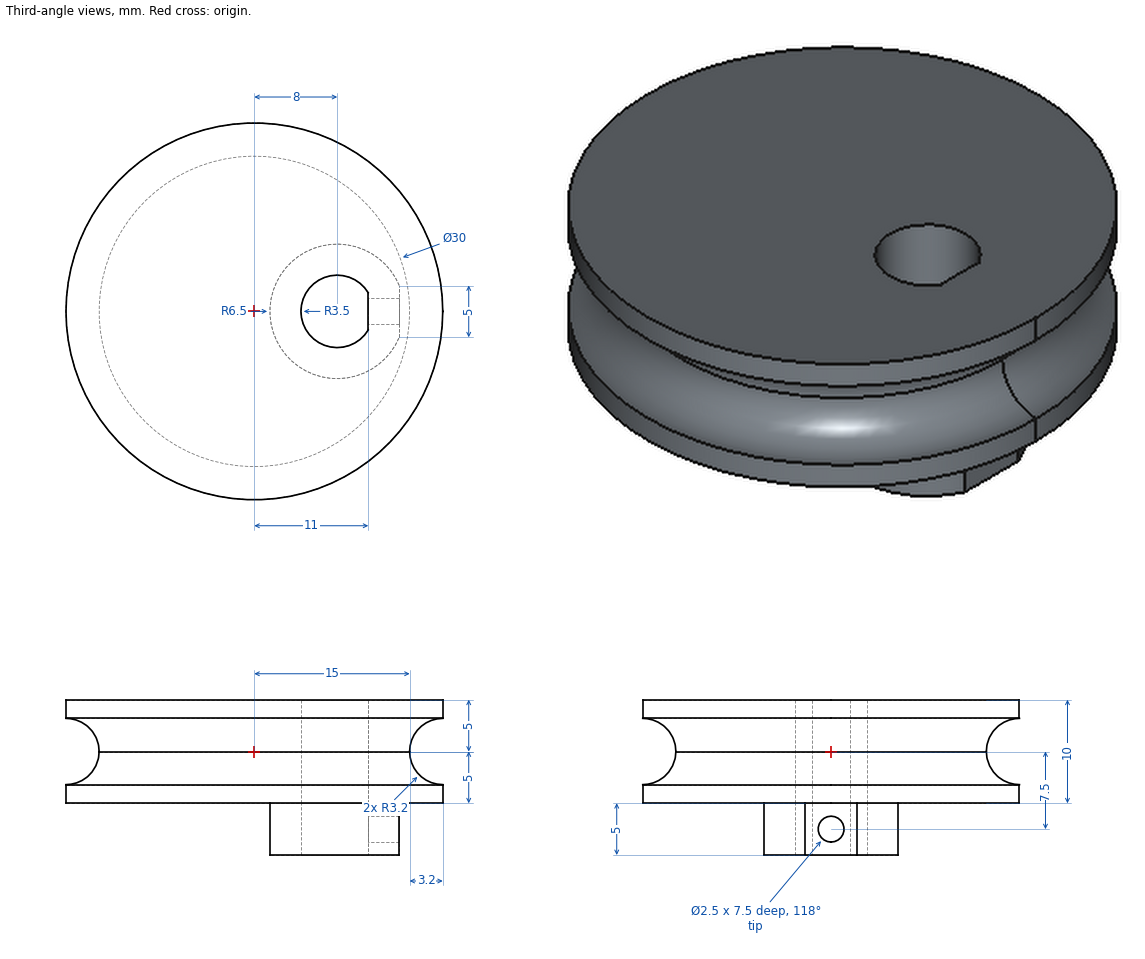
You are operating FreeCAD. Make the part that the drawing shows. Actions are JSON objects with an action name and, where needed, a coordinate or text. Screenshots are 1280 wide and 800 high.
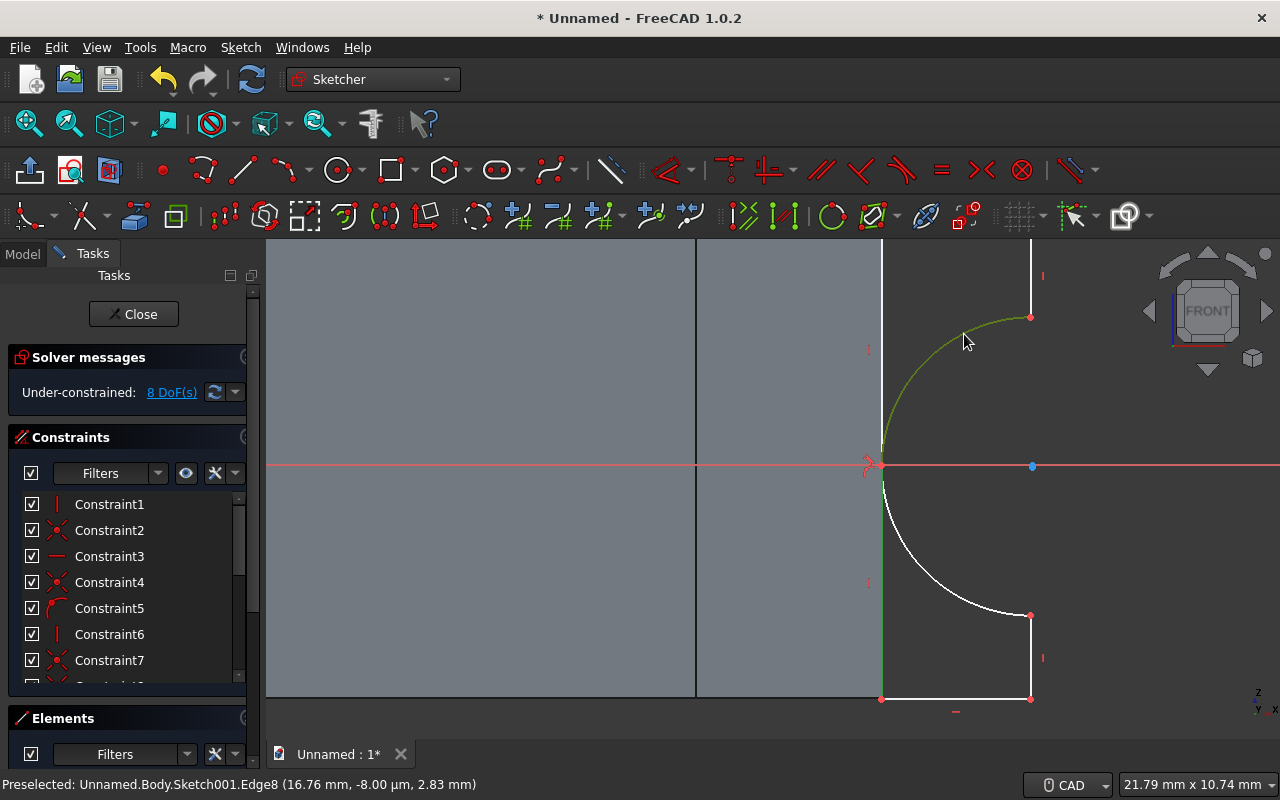
{"action": "left_click", "coordinate": [902, 170]}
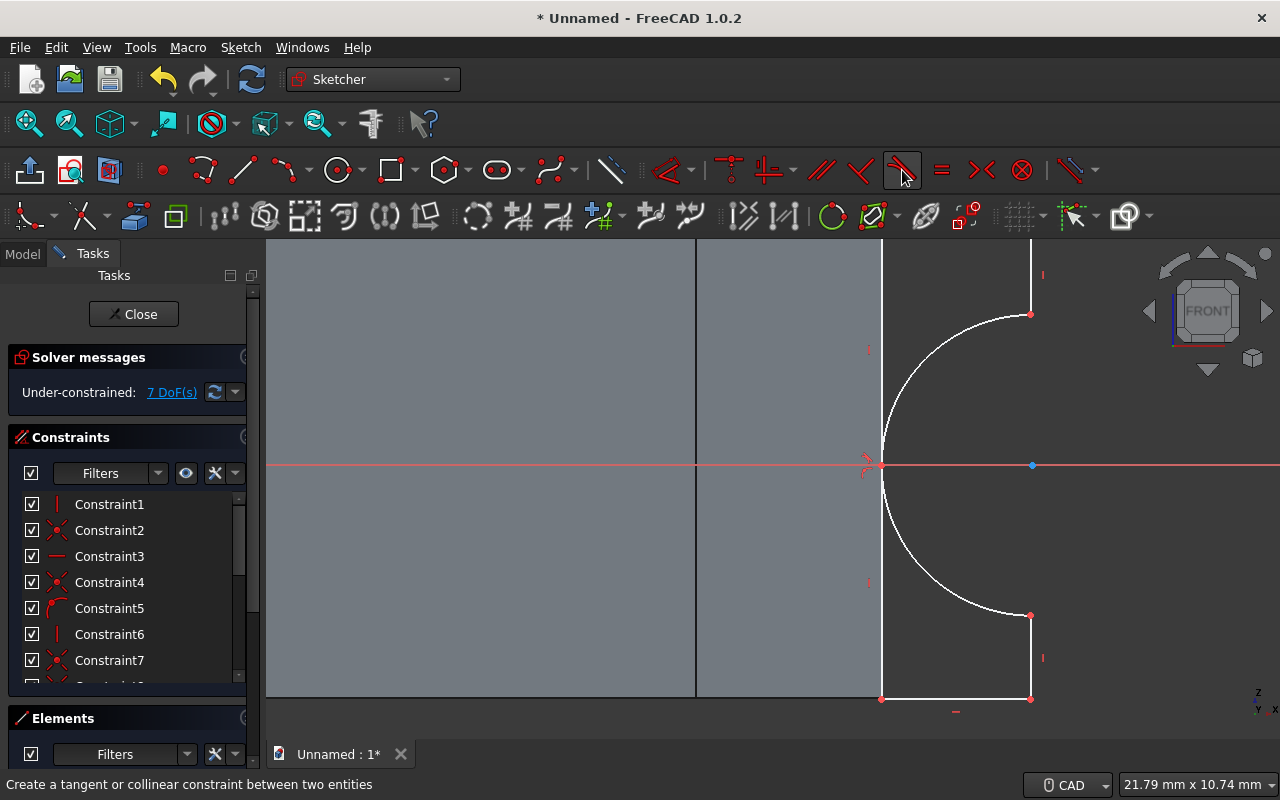
{"action": "left_click", "coordinate": [898, 533]}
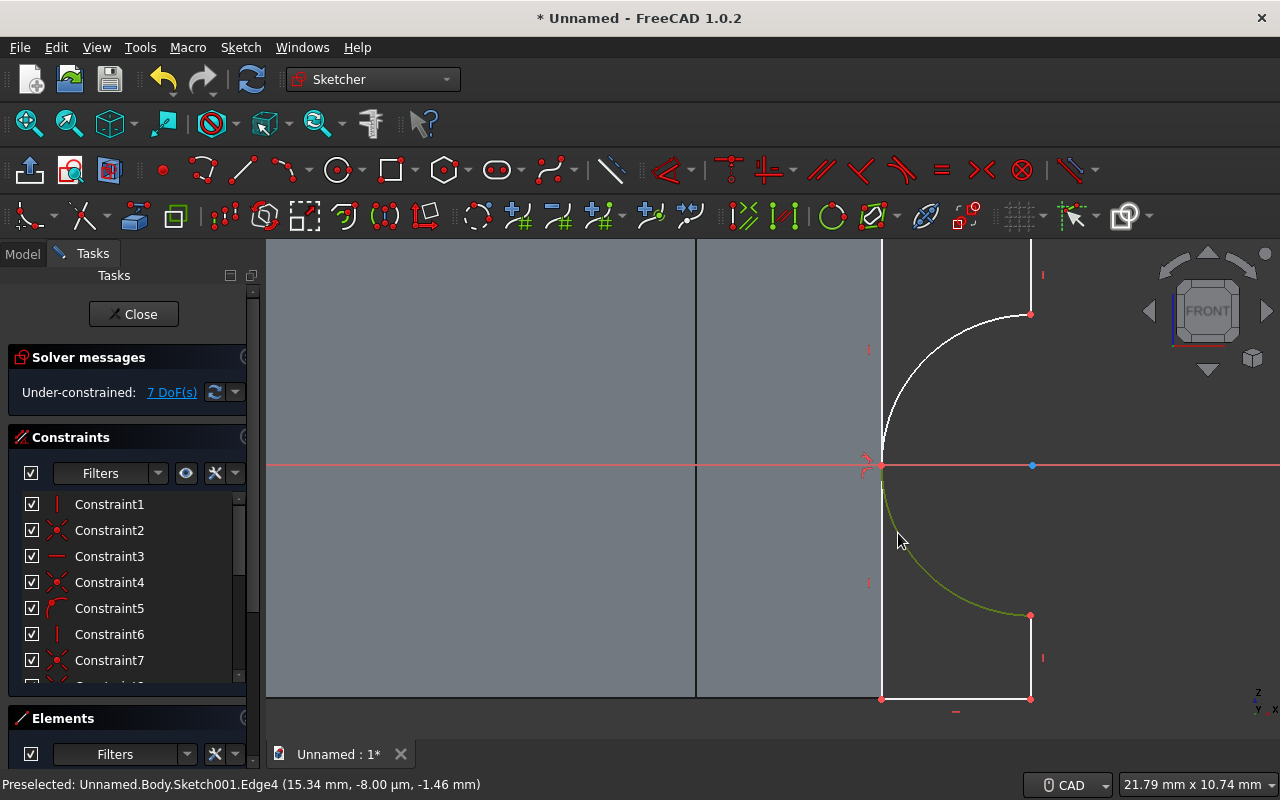
{"action": "left_click", "coordinate": [963, 332]}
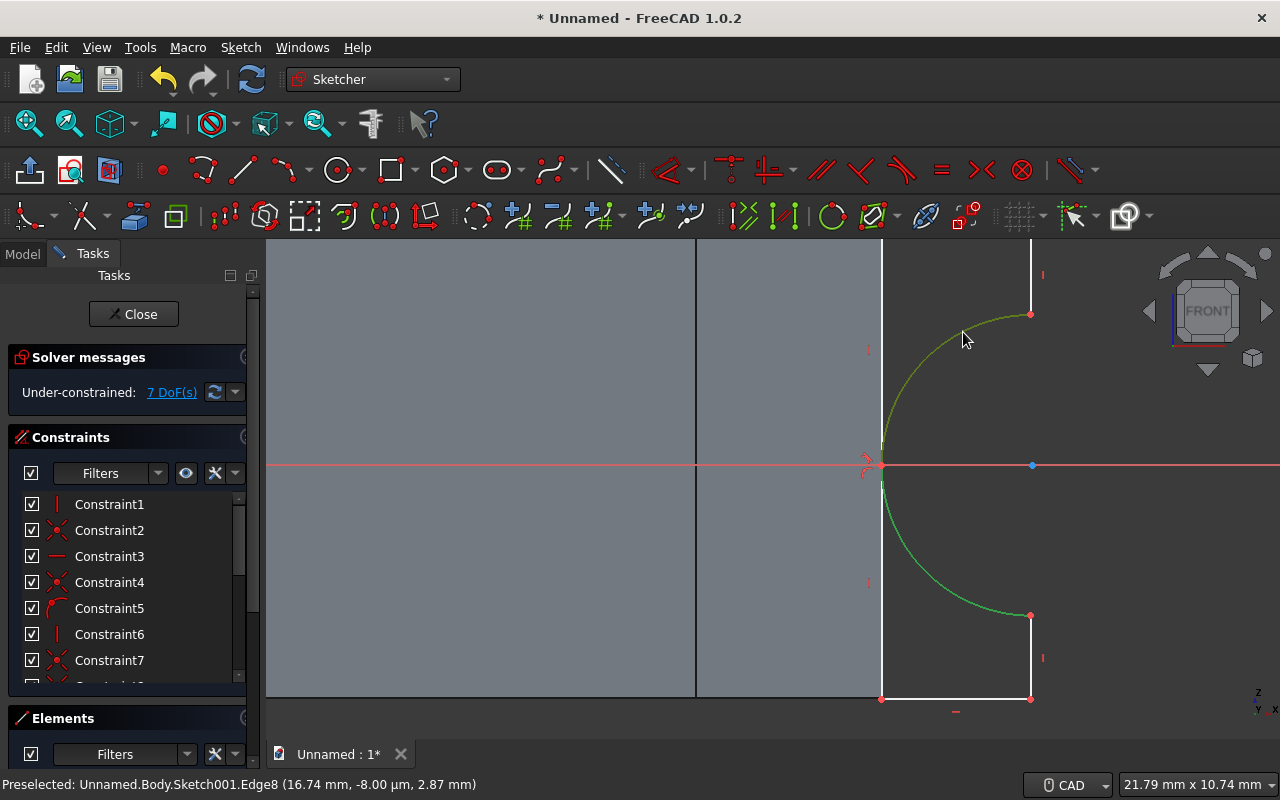
{"action": "left_click", "coordinate": [942, 170]}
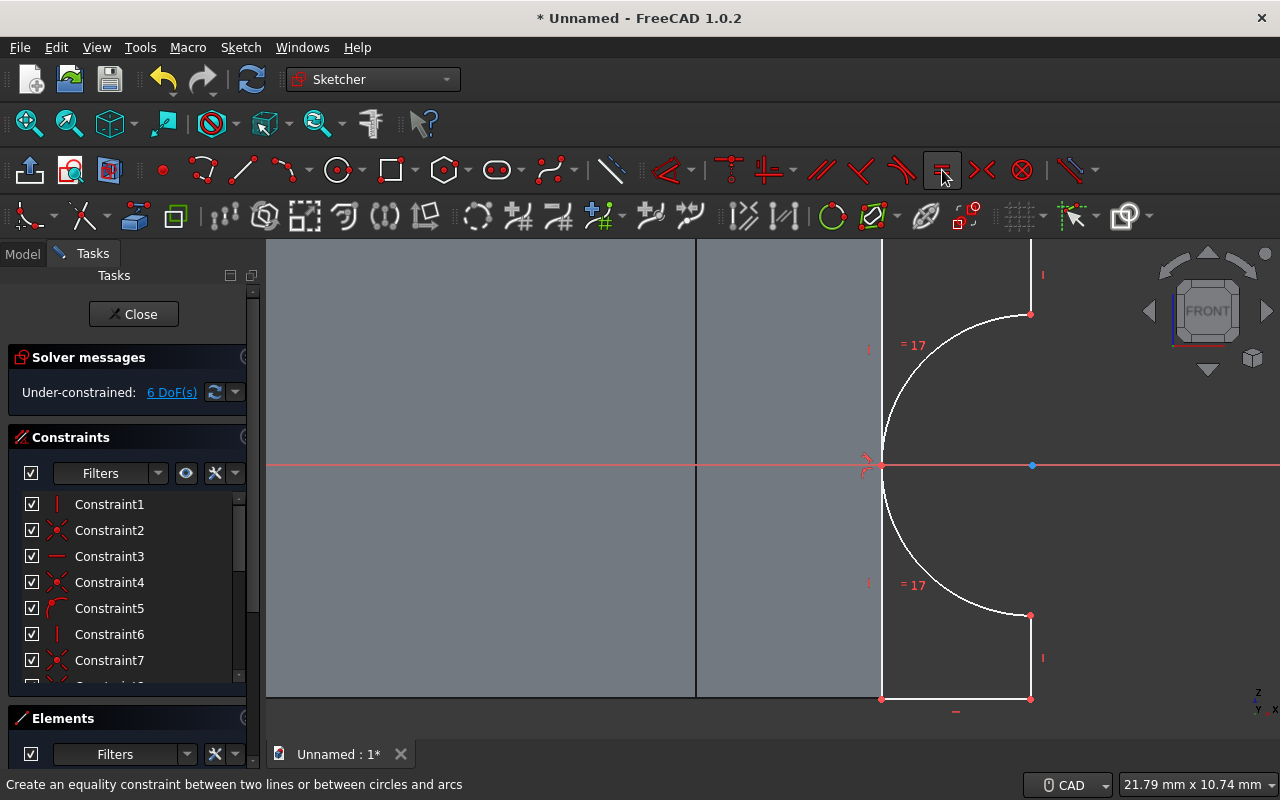
{"action": "left_click", "coordinate": [666, 170]}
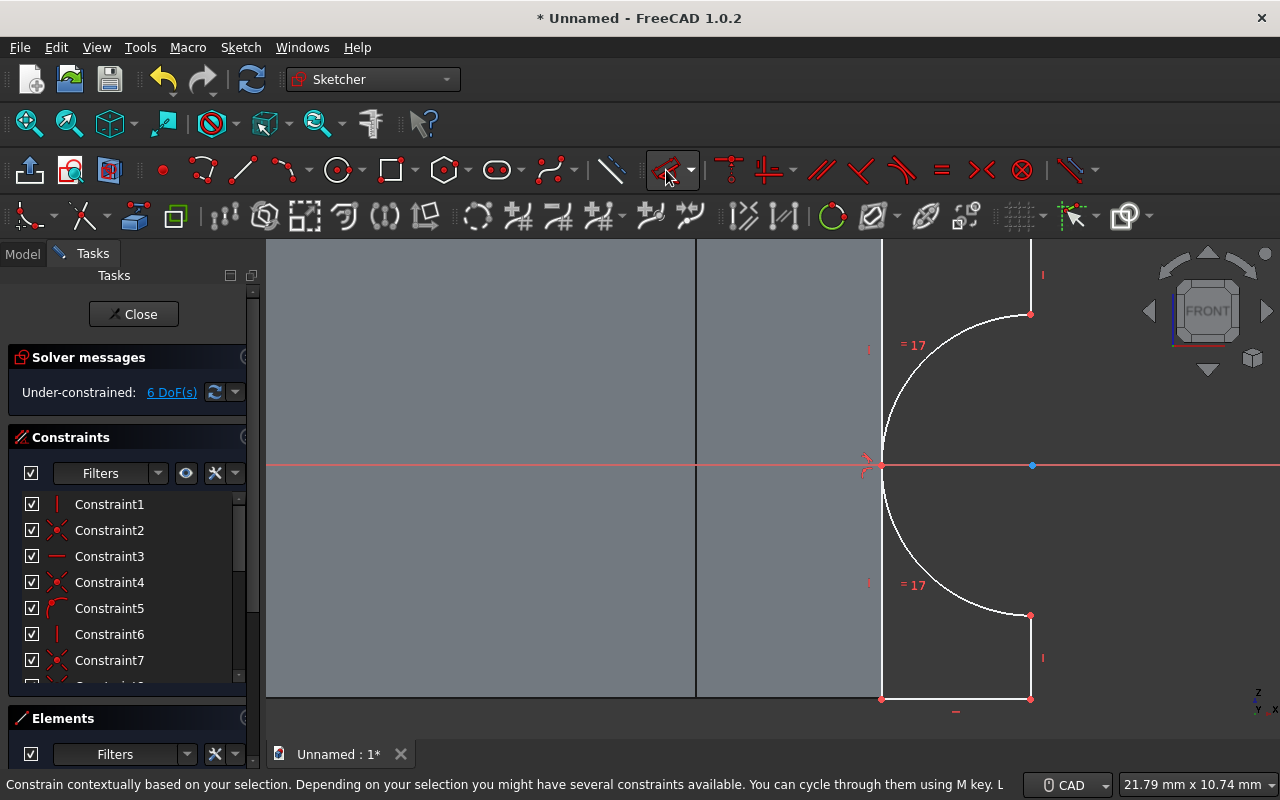
{"action": "left_click", "coordinate": [898, 533]}
{"action": "left_click", "coordinate": [929, 615]}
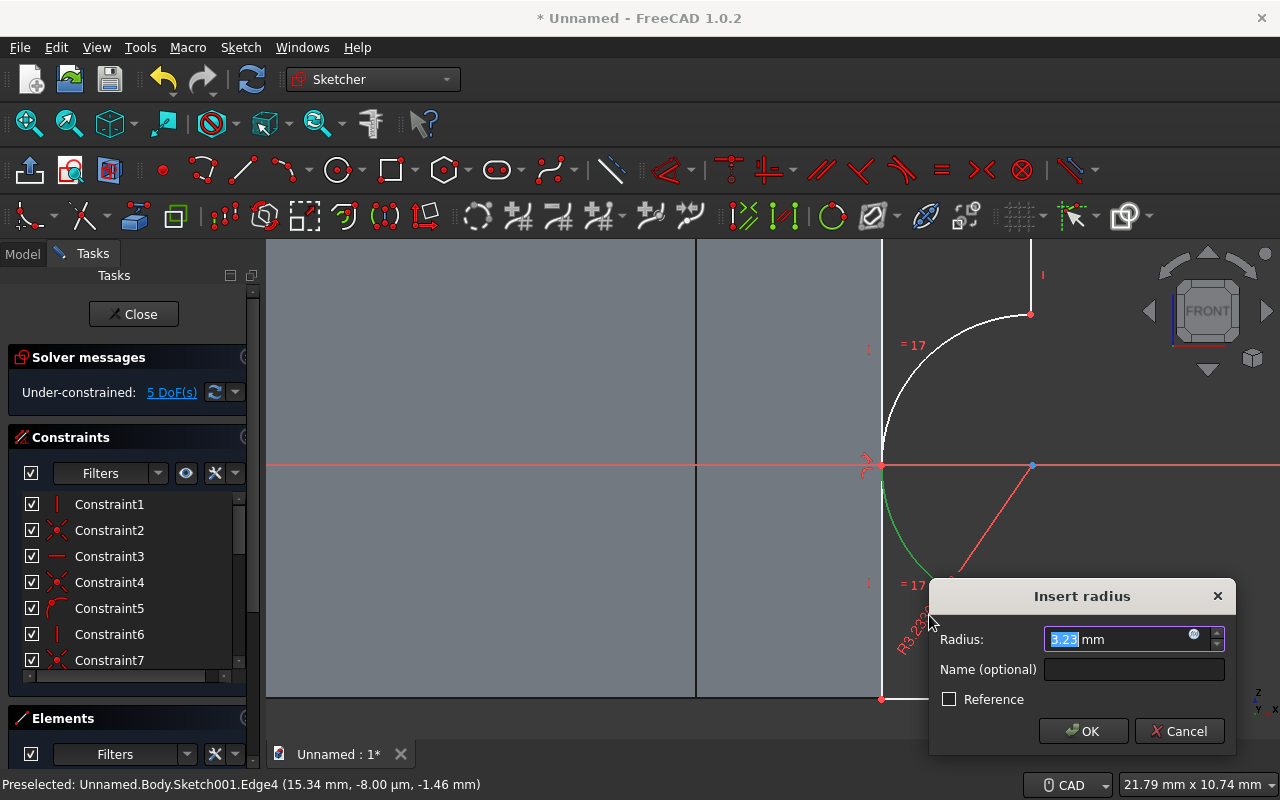
{"action": "type", "text": "3.2"}
{"action": "key", "text": "Return"}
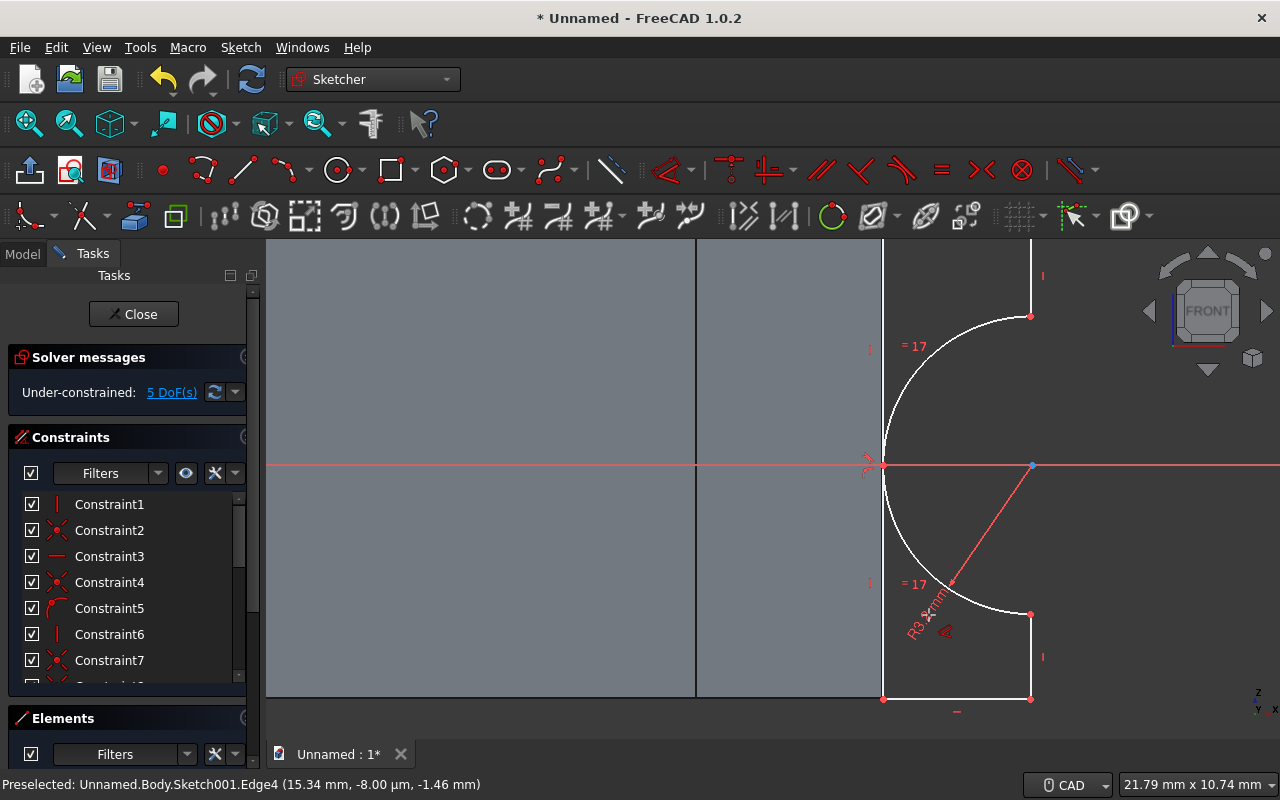
{"action": "left_click", "coordinate": [883, 629]}
{"action": "left_click", "coordinate": [917, 582]}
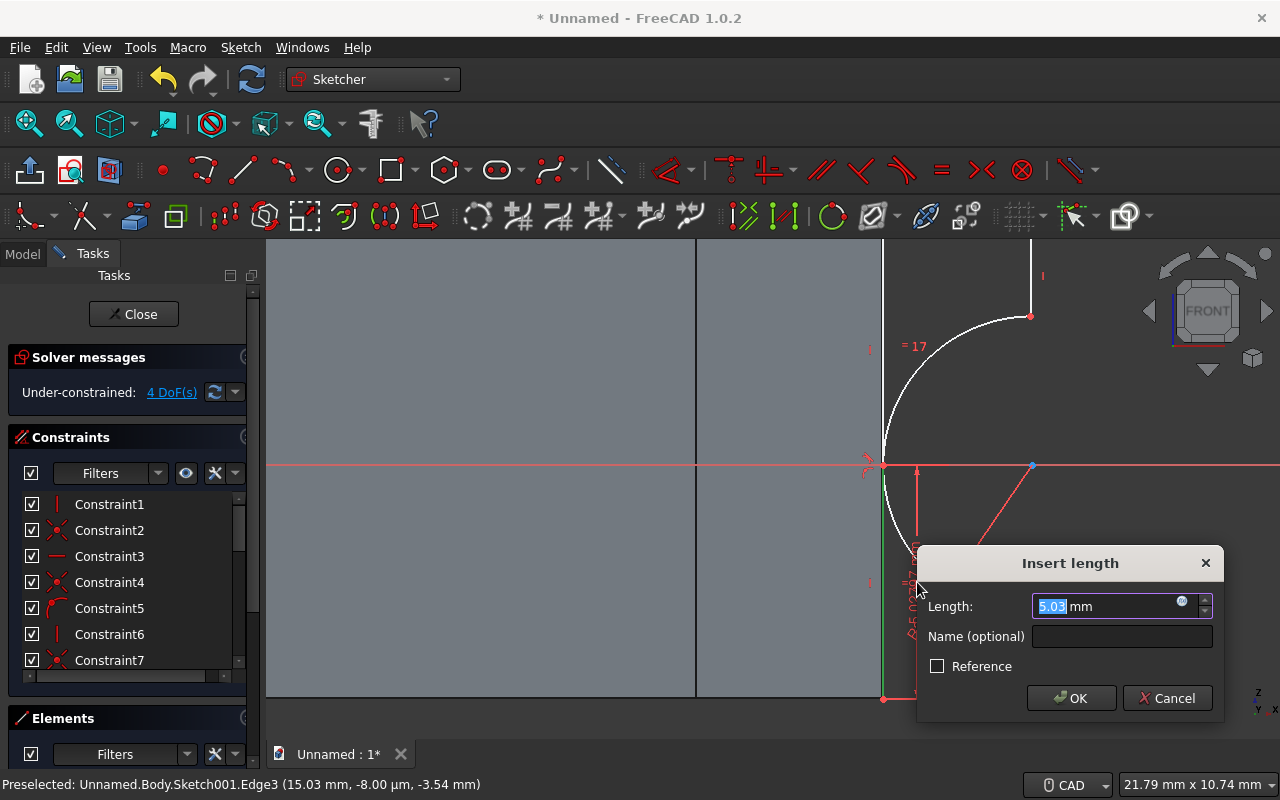
{"action": "type", "text": "5"}
{"action": "key", "text": "Return"}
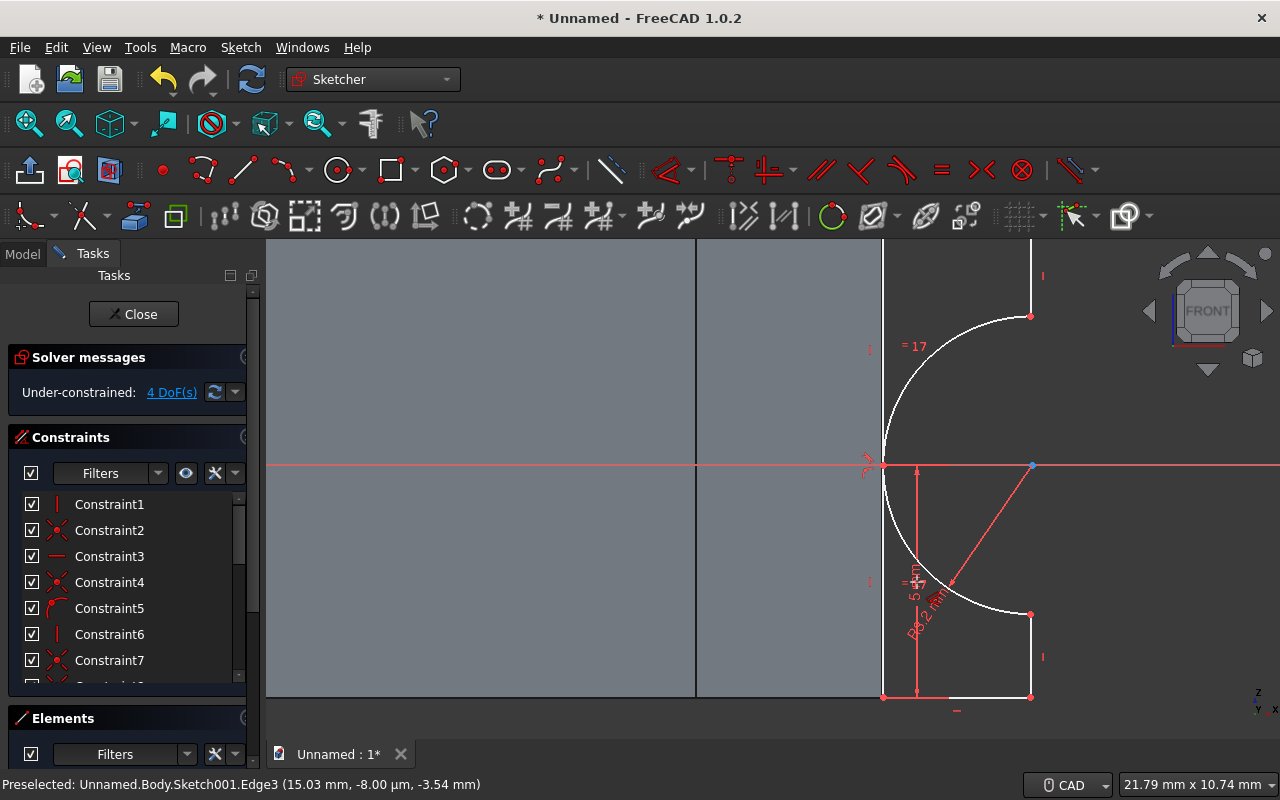
{"action": "left_click", "coordinate": [883, 396]}
{"action": "left_click", "coordinate": [917, 321]}